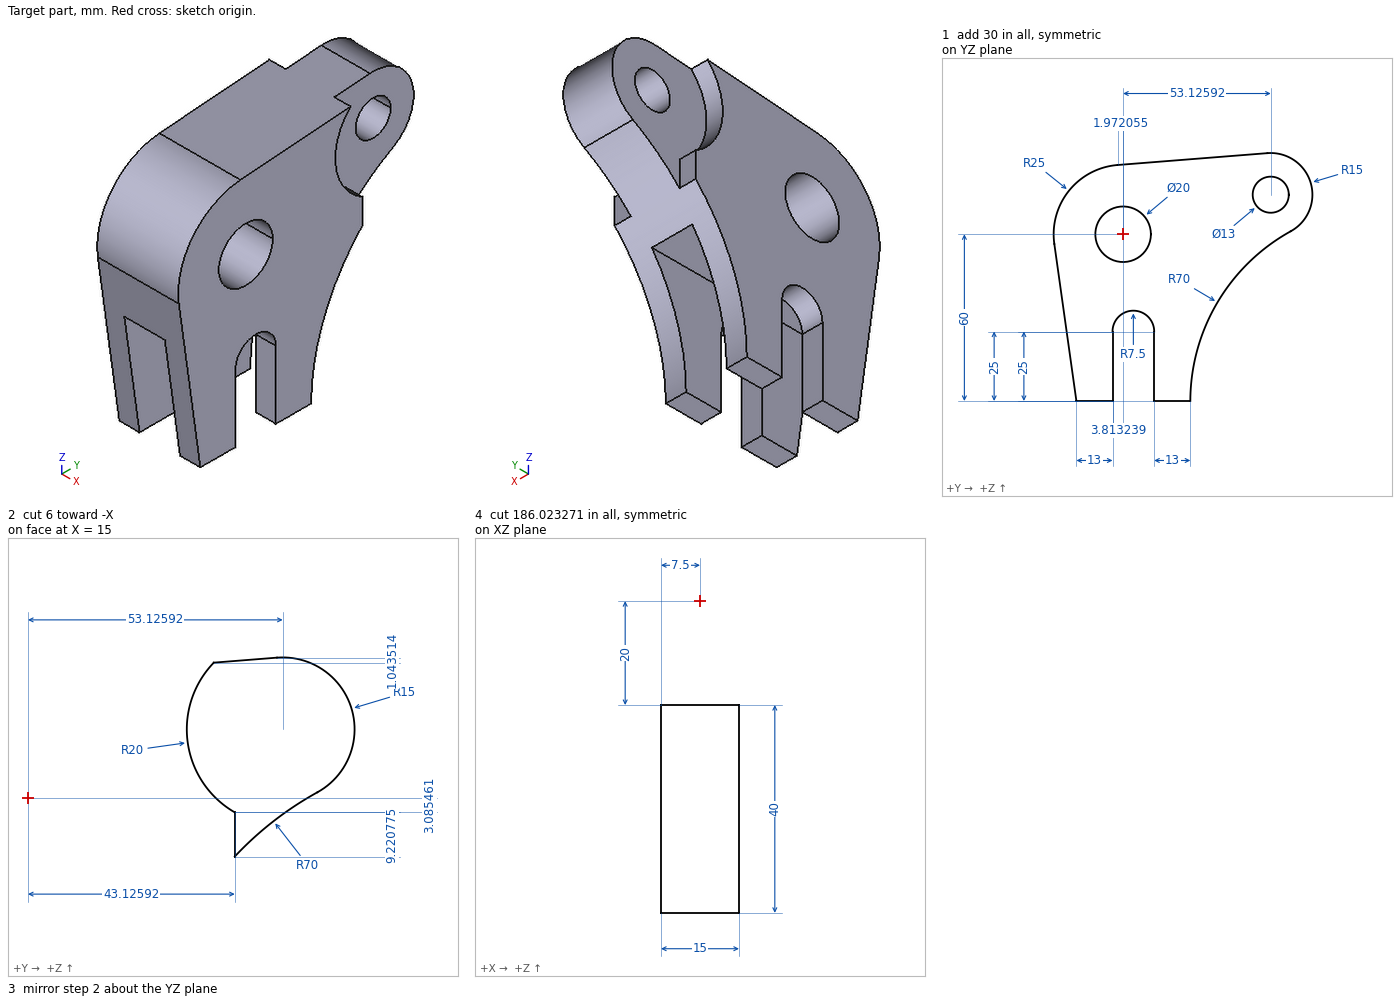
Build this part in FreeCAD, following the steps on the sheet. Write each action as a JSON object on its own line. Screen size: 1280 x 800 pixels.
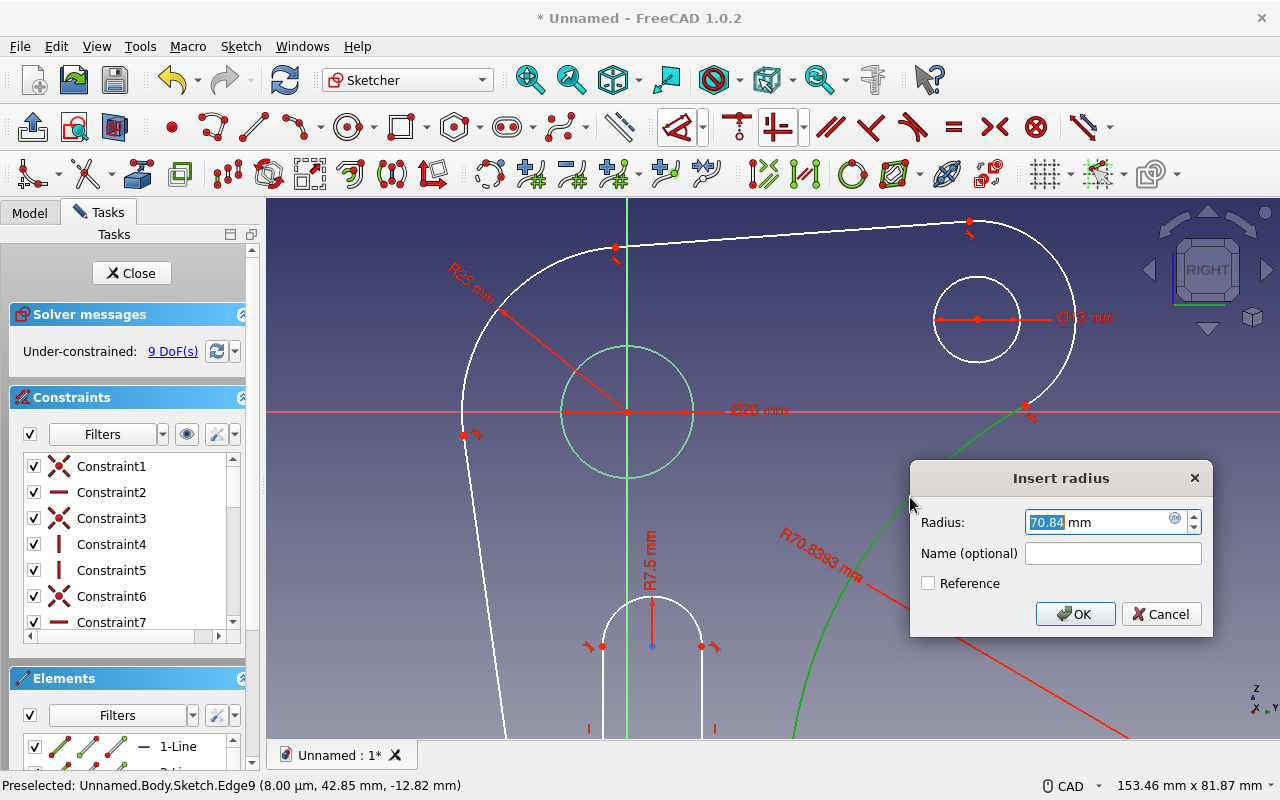
{"action": "type", "text": "70"}
{"action": "key", "text": "Return"}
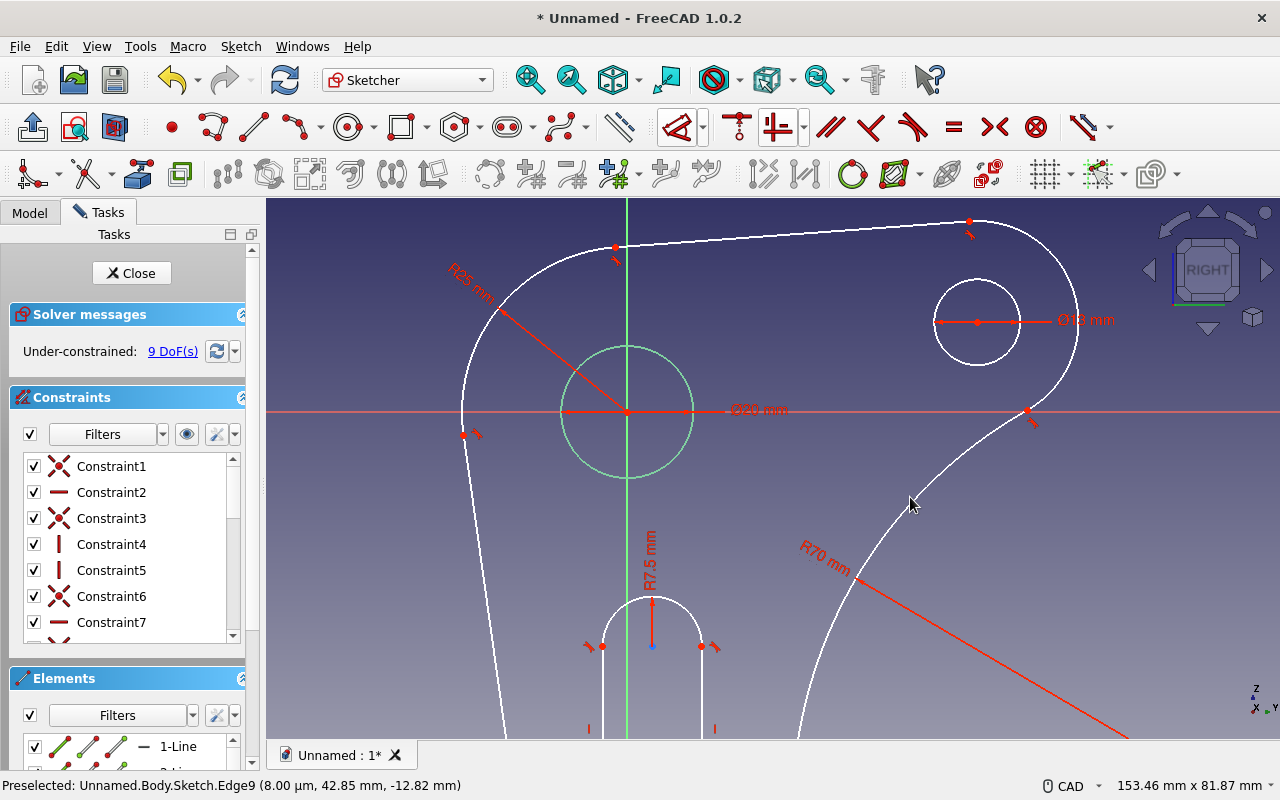
{"action": "left_click", "coordinate": [1075, 347]}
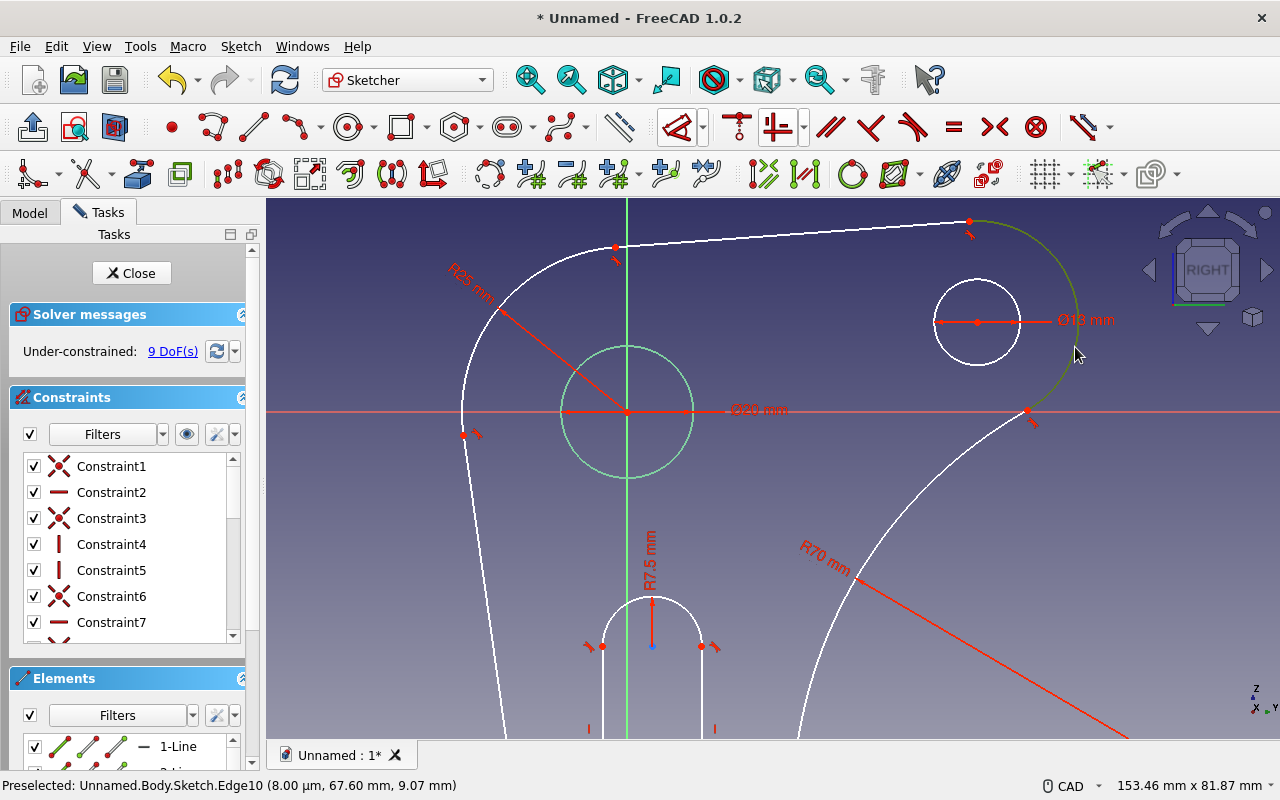
{"action": "key", "text": "k r"}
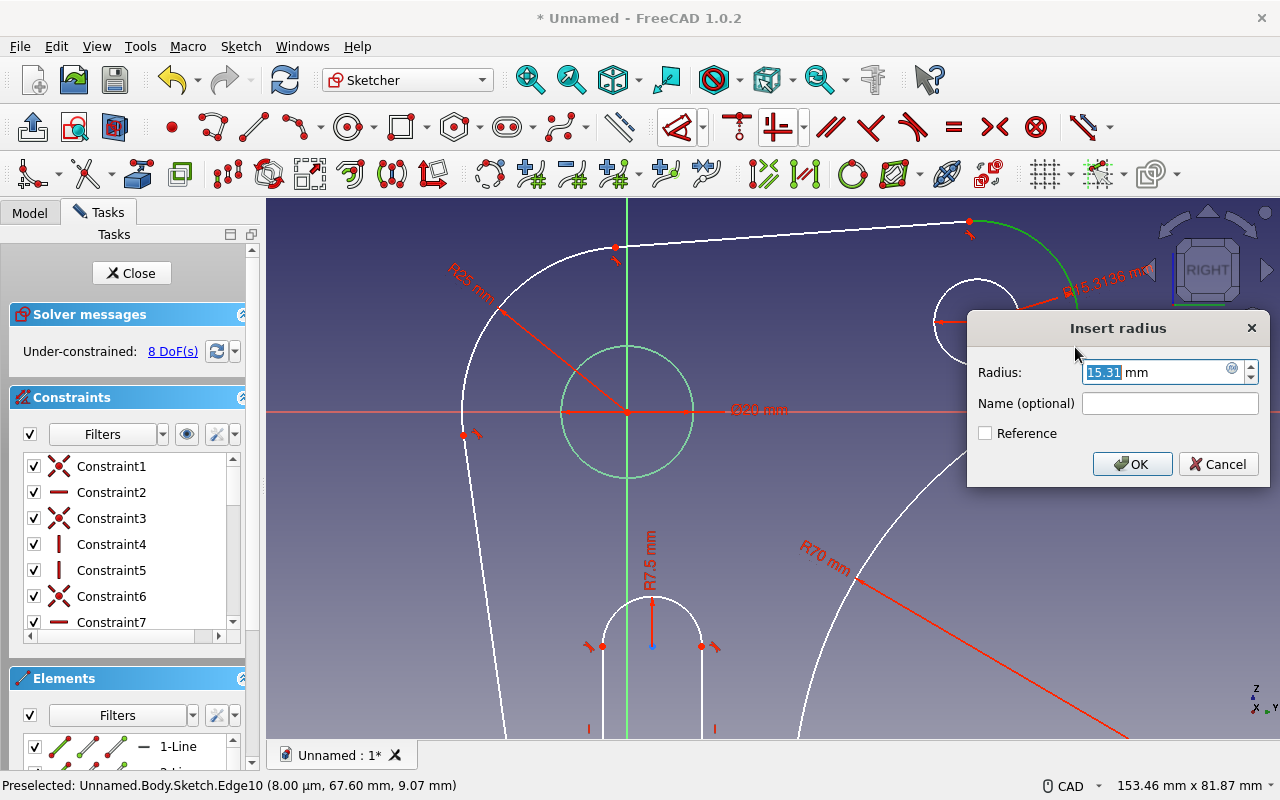
{"action": "type", "text": "15"}
{"action": "key", "text": "Return"}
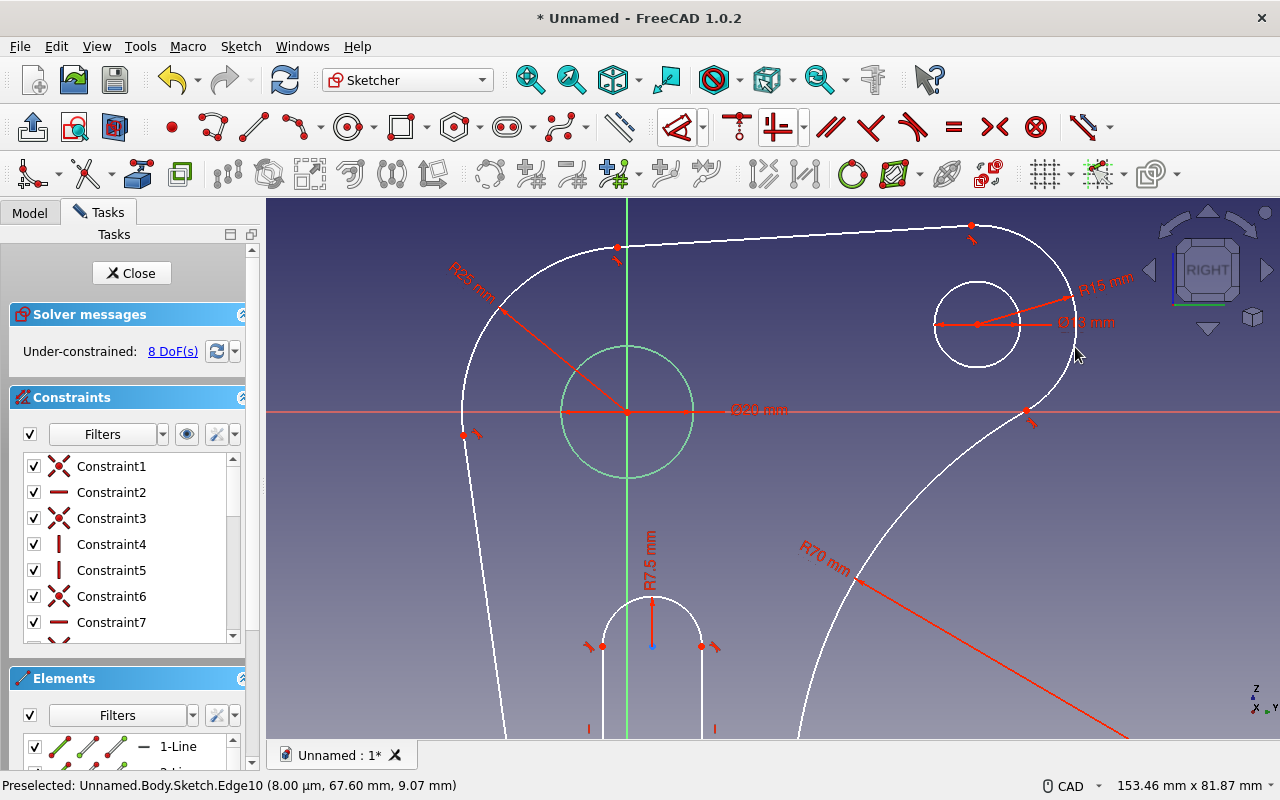
{"action": "scroll", "coordinate": [627, 413], "scroll_direction": "down", "scroll_amount": 3}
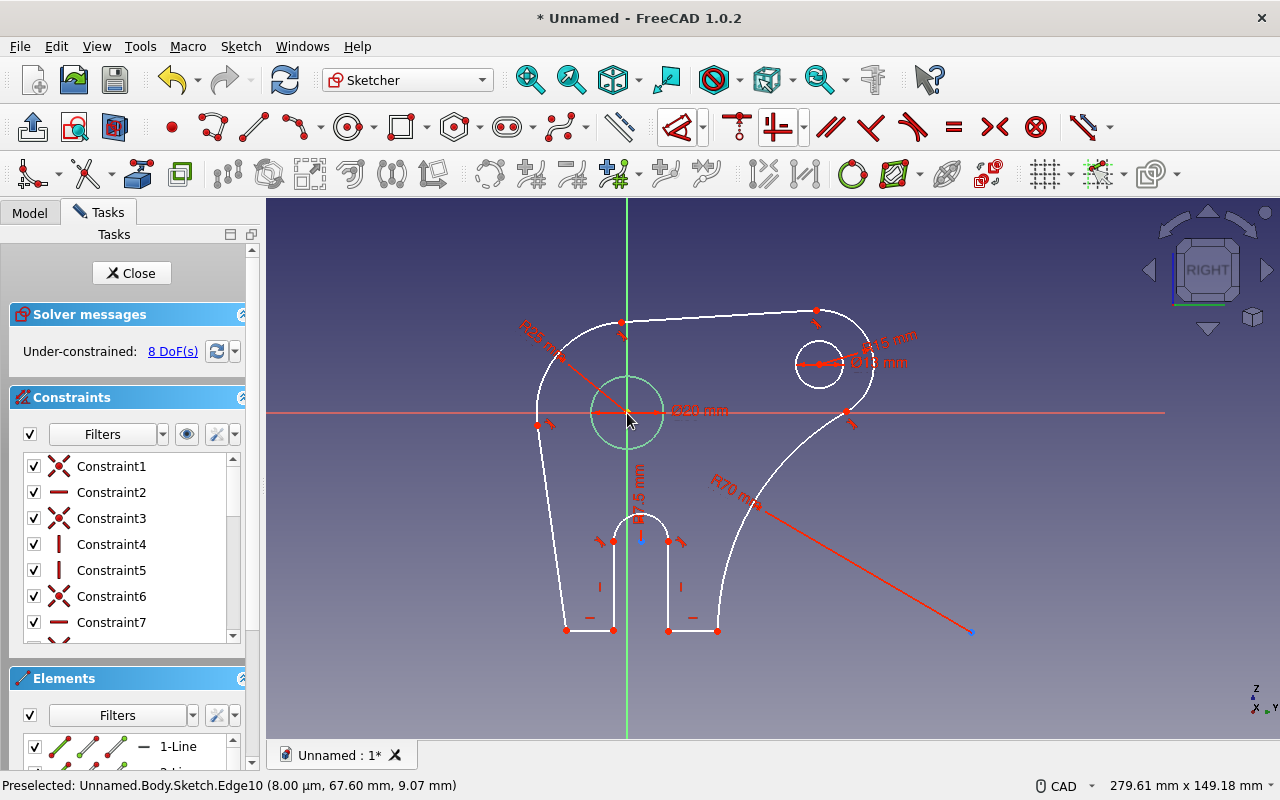
{"action": "left_click", "coordinate": [581, 631]}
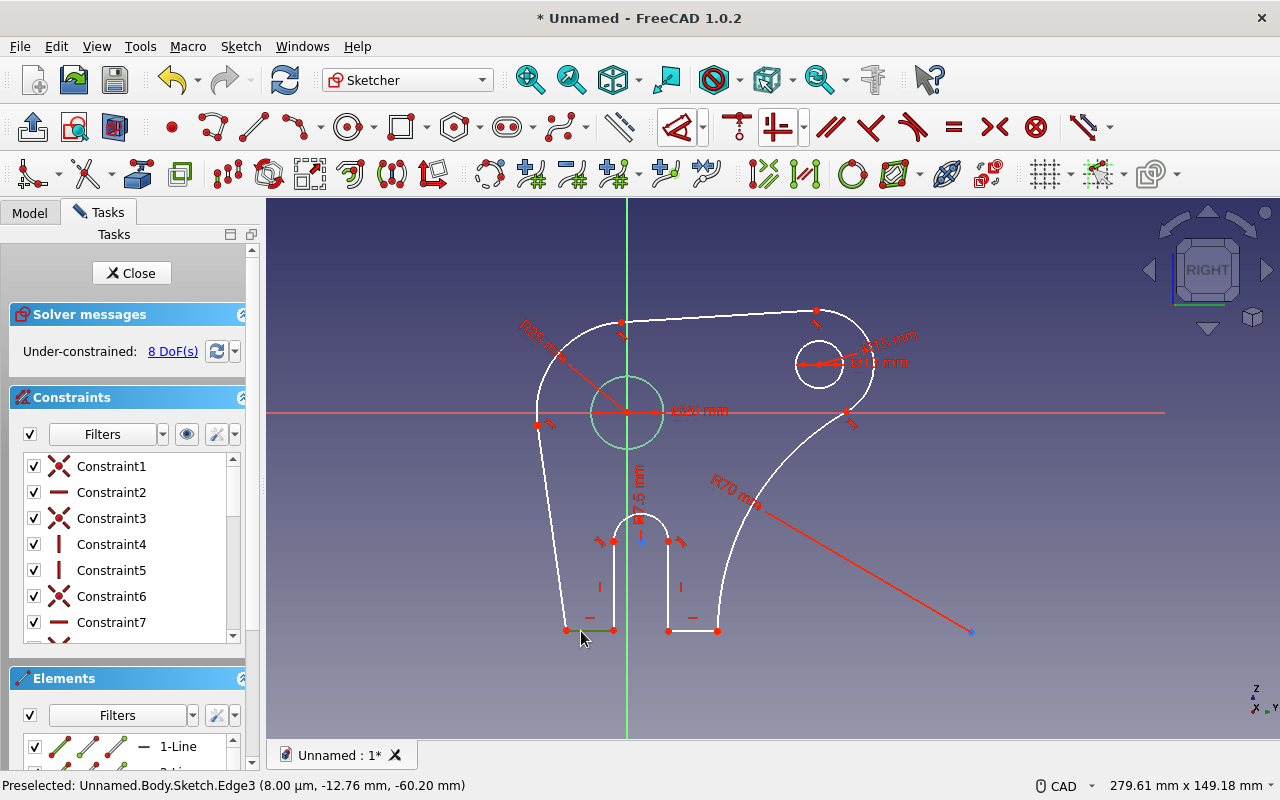
{"action": "key", "text": "l"}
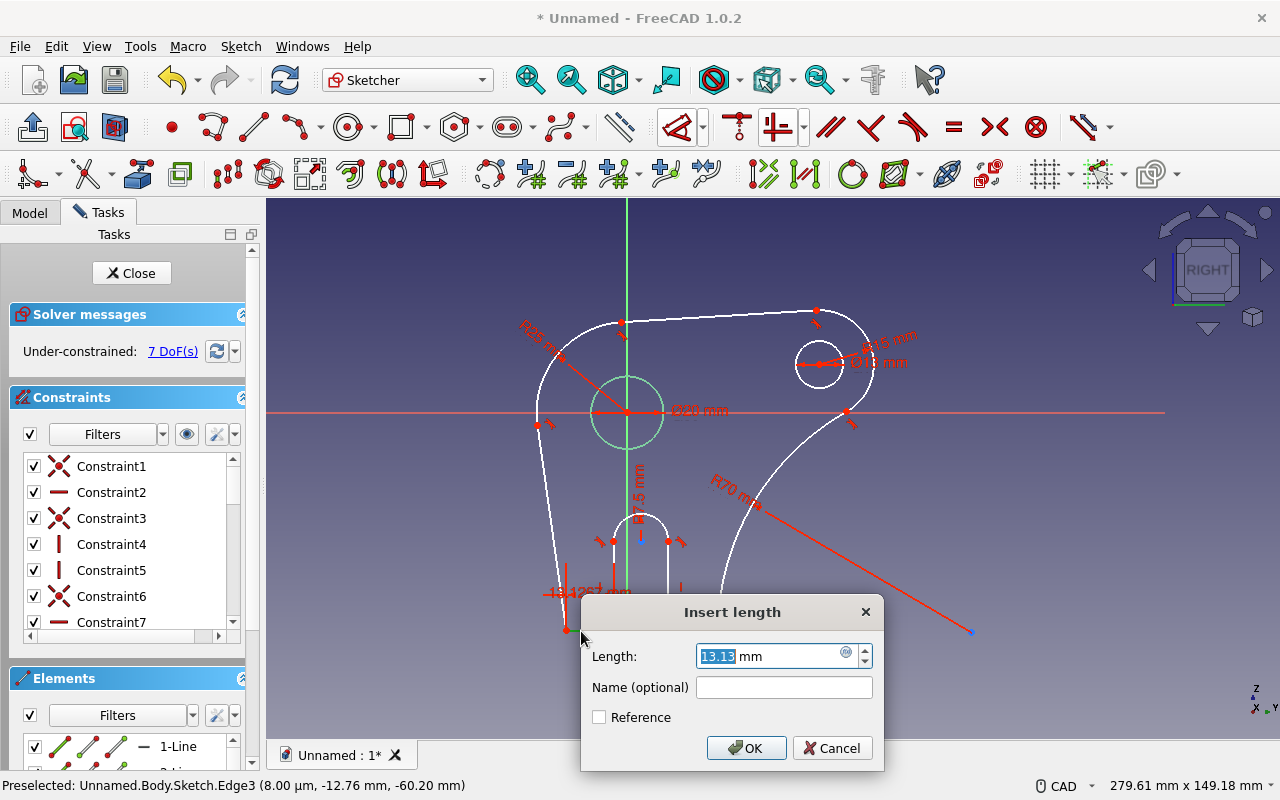
{"action": "type", "text": "13"}
{"action": "key", "text": "Return"}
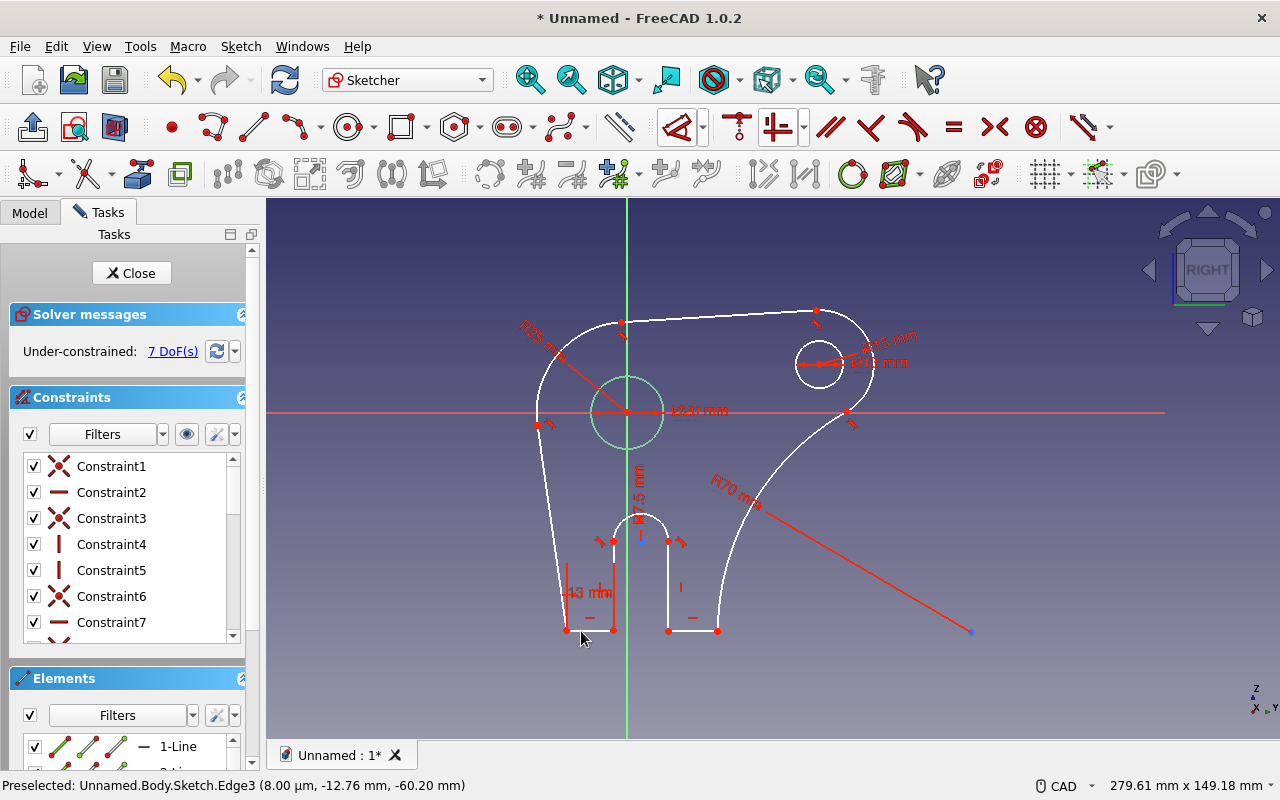
{"action": "left_click", "coordinate": [614, 604]}